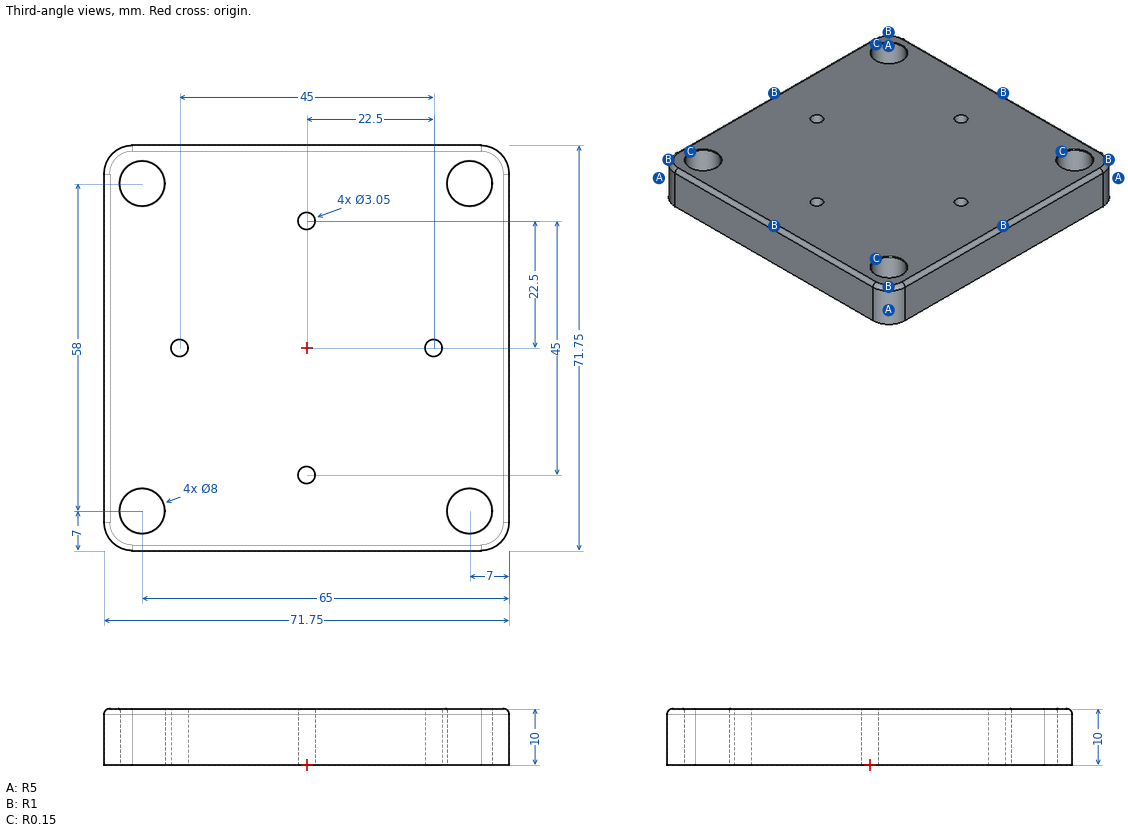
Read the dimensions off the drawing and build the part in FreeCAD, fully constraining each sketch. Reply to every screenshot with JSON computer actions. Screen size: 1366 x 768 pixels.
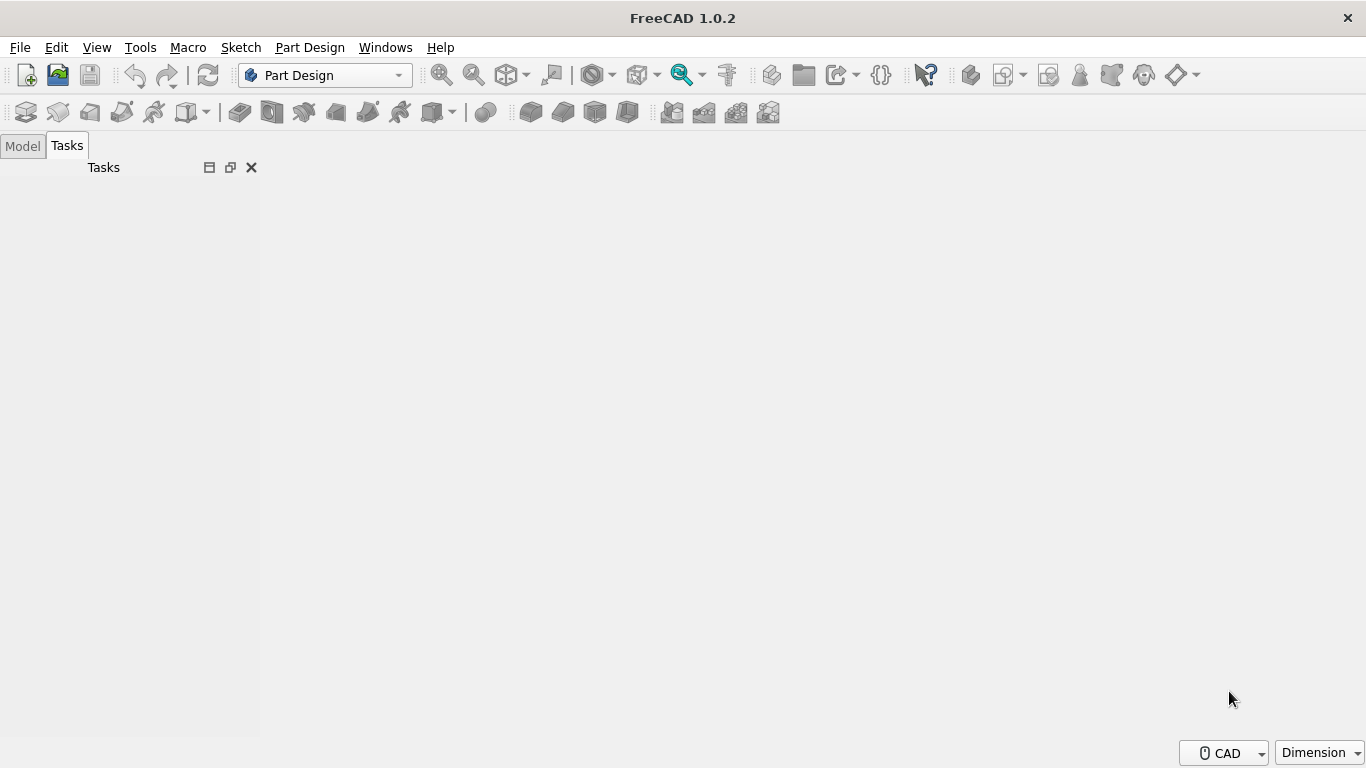
{"action": "left_click", "coordinate": [26, 76]}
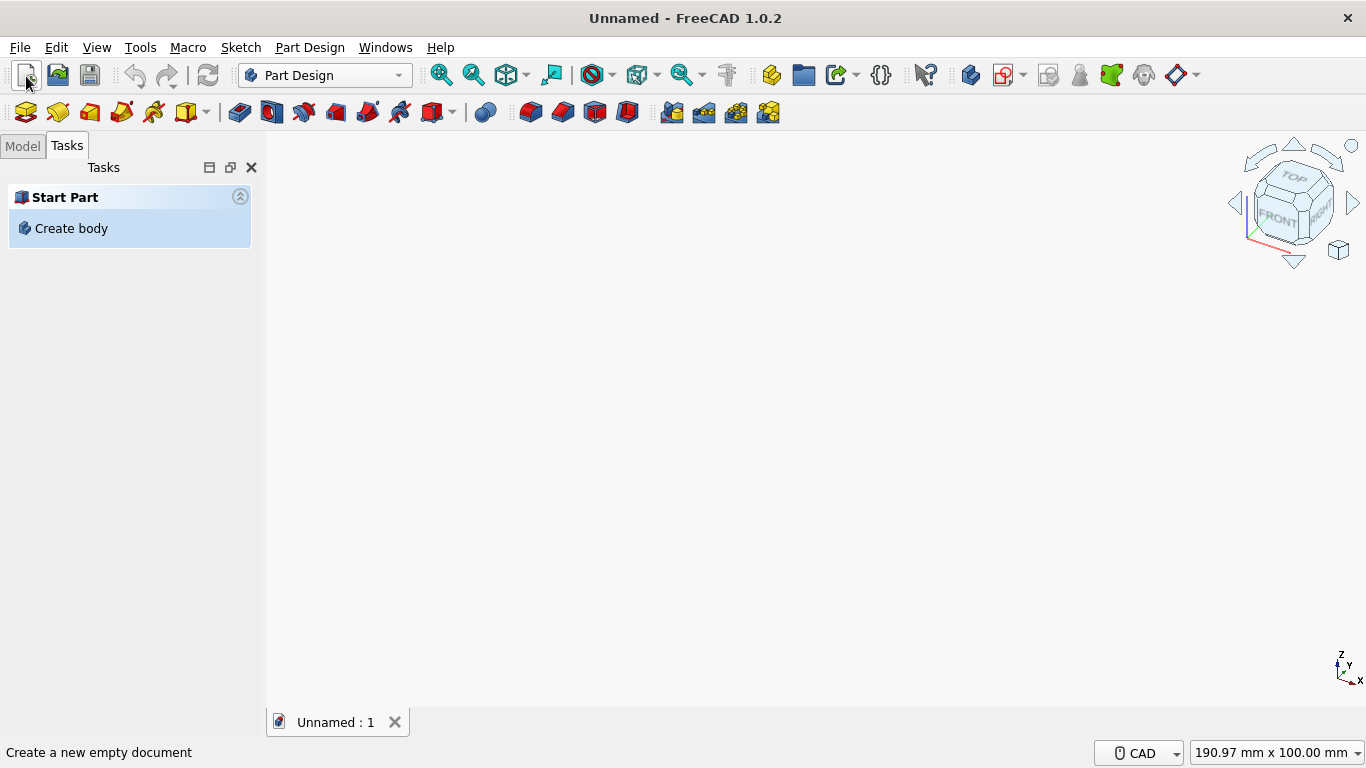
{"action": "left_click", "coordinate": [1004, 76]}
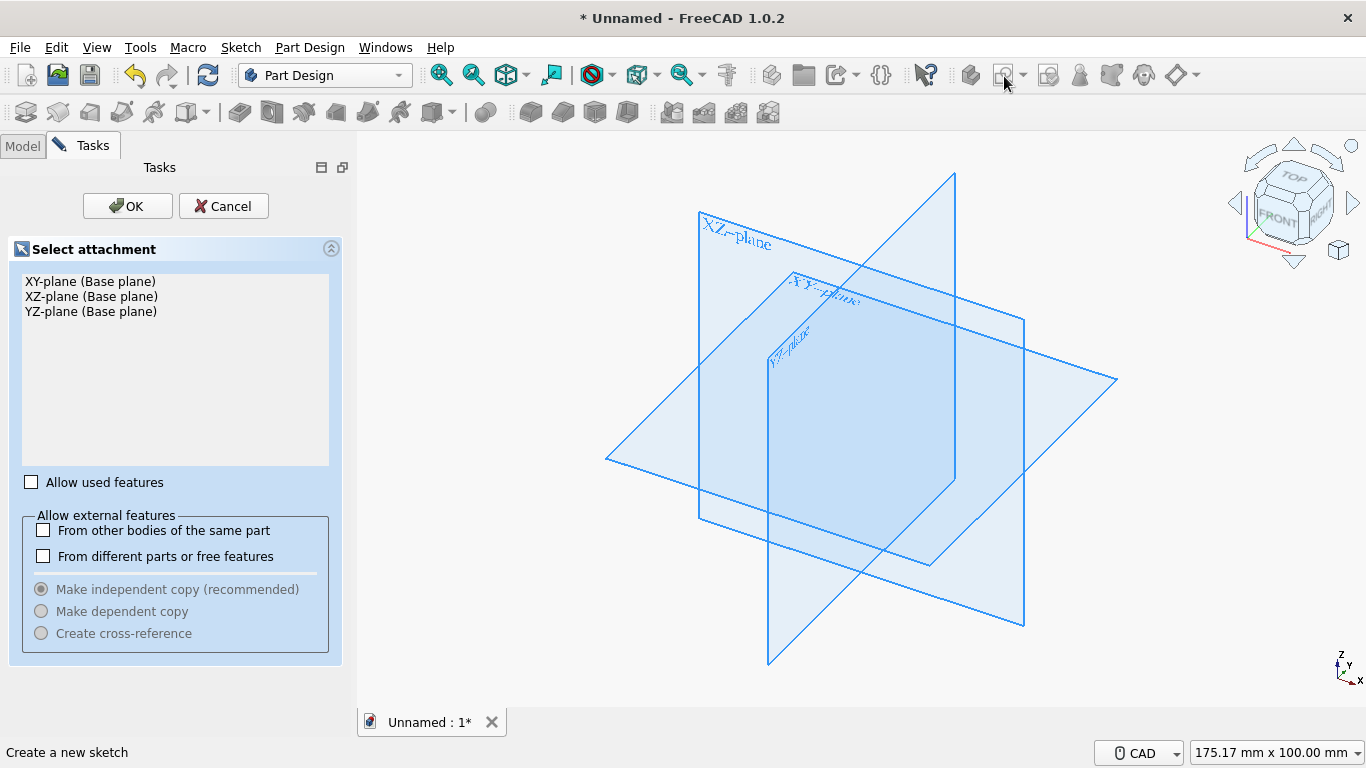
{"action": "left_click", "coordinate": [82, 282]}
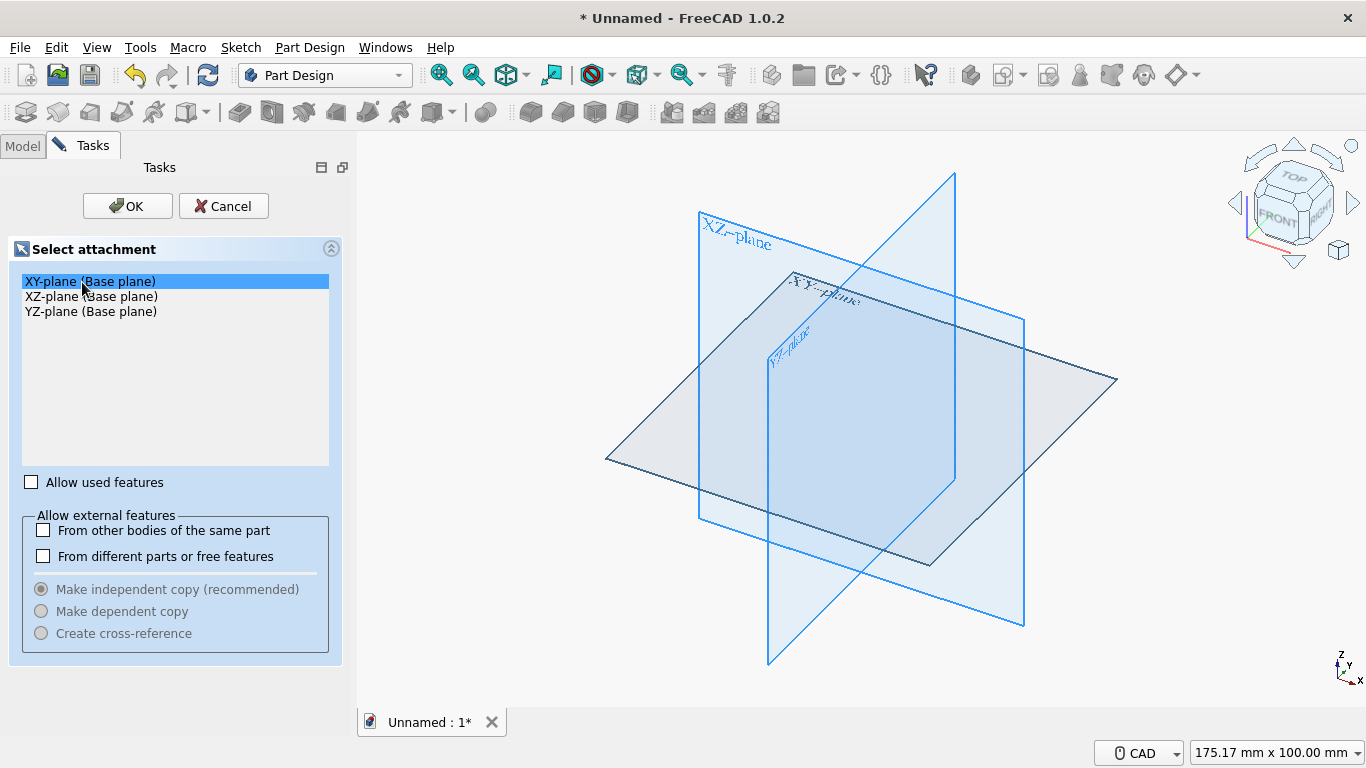
{"action": "left_click", "coordinate": [128, 206]}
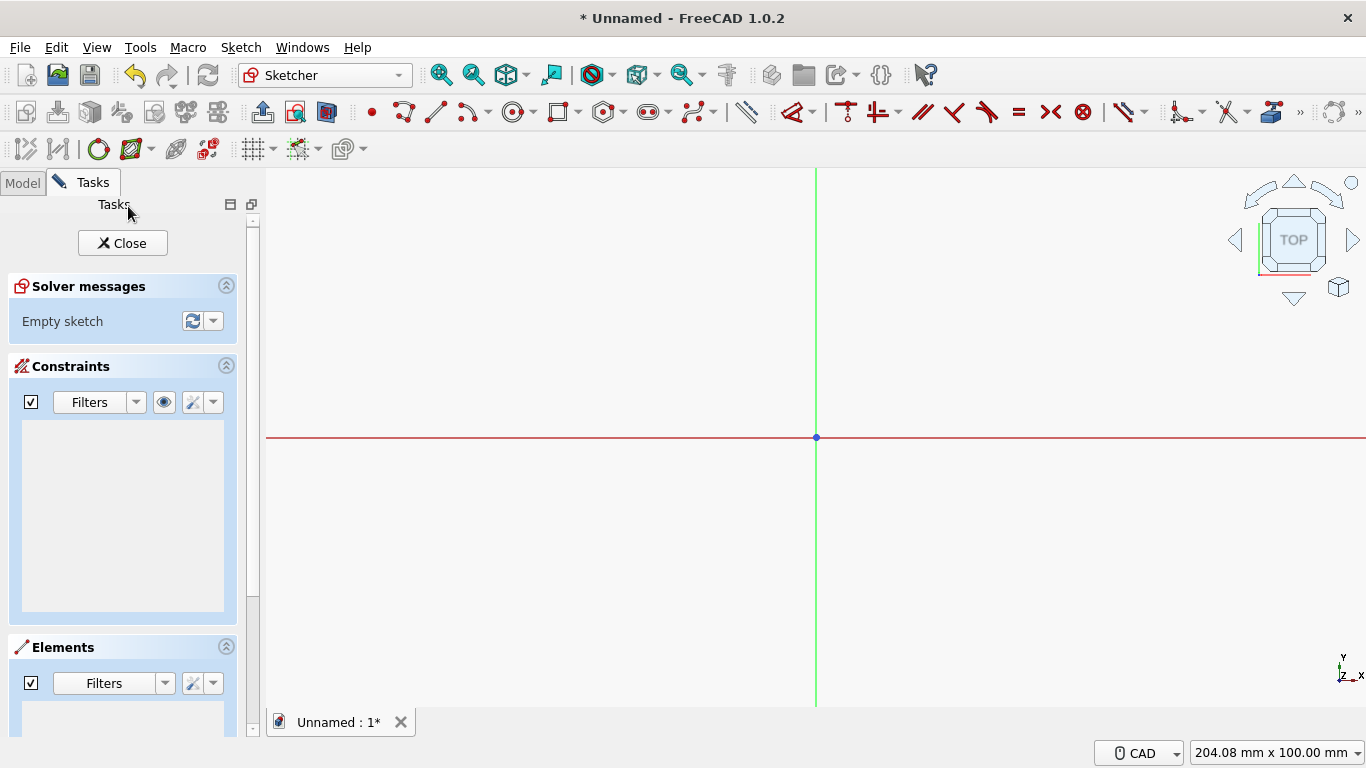
{"action": "key", "text": "g v"}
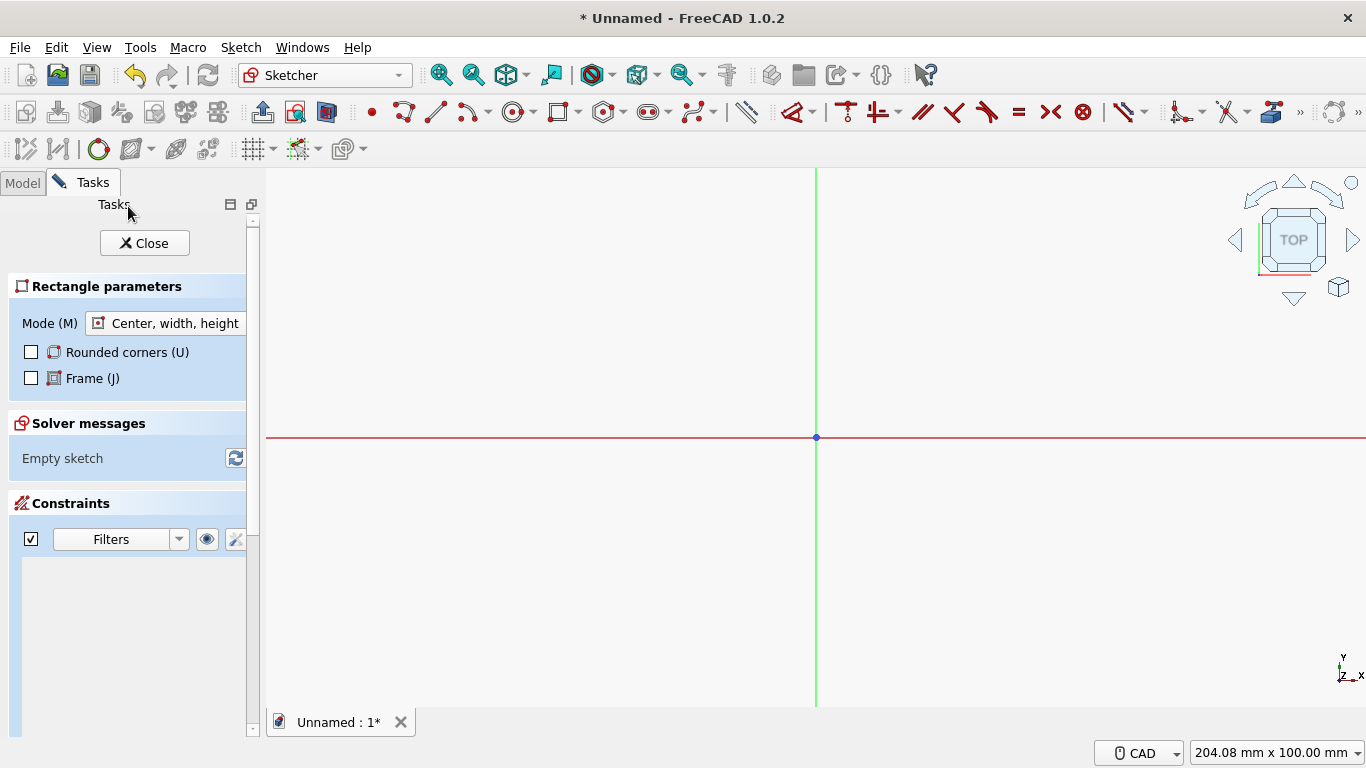
{"action": "left_click", "coordinate": [816, 438]}
{"action": "left_click", "coordinate": [1009, 244]}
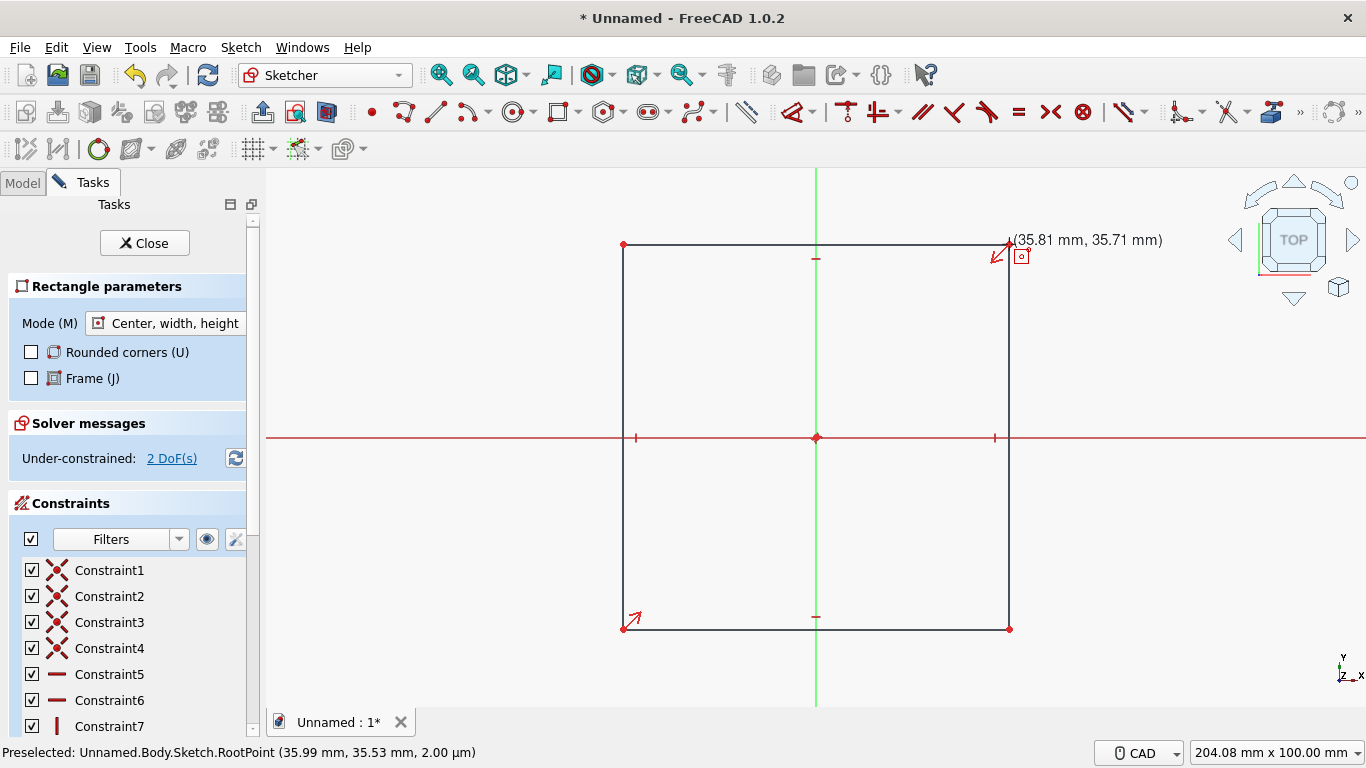
{"action": "left_click", "coordinate": [514, 112]}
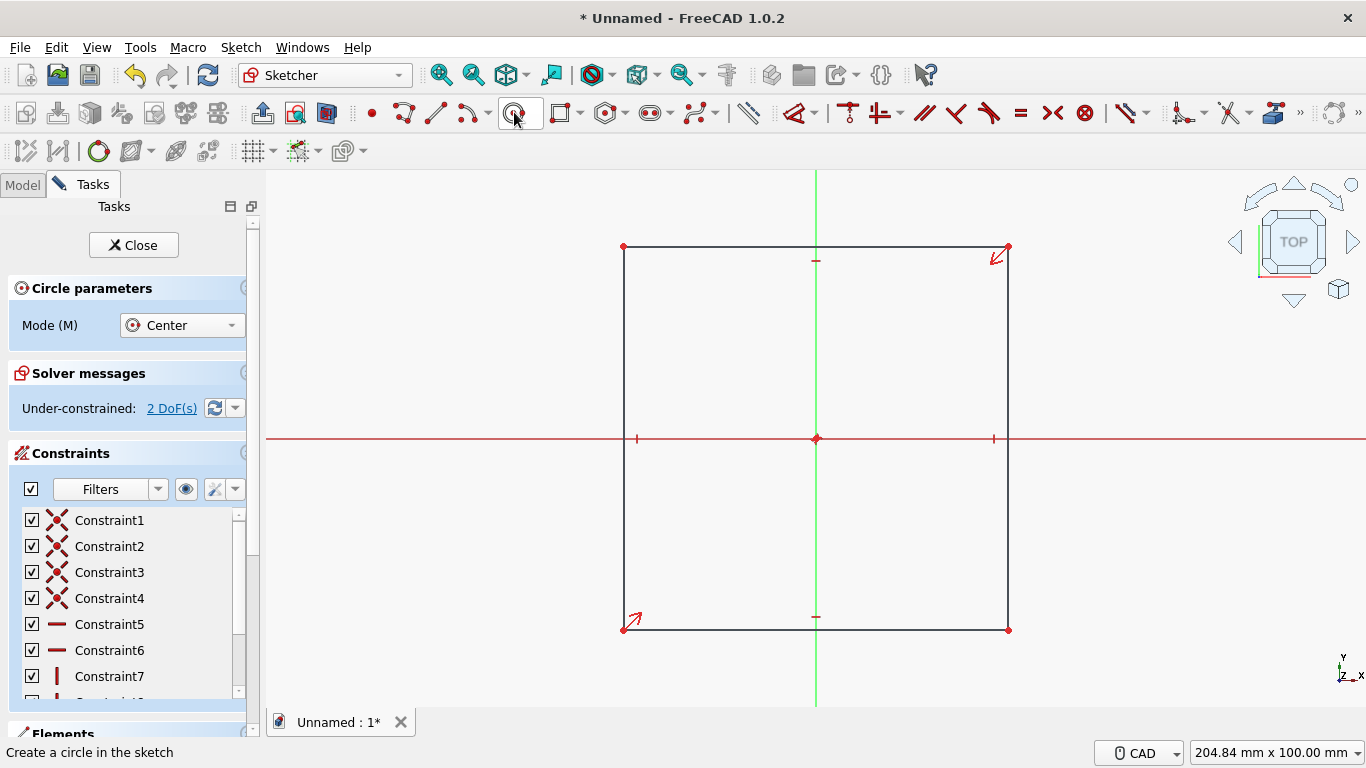
{"action": "left_click", "coordinate": [660, 594]}
{"action": "left_click", "coordinate": [675, 578]}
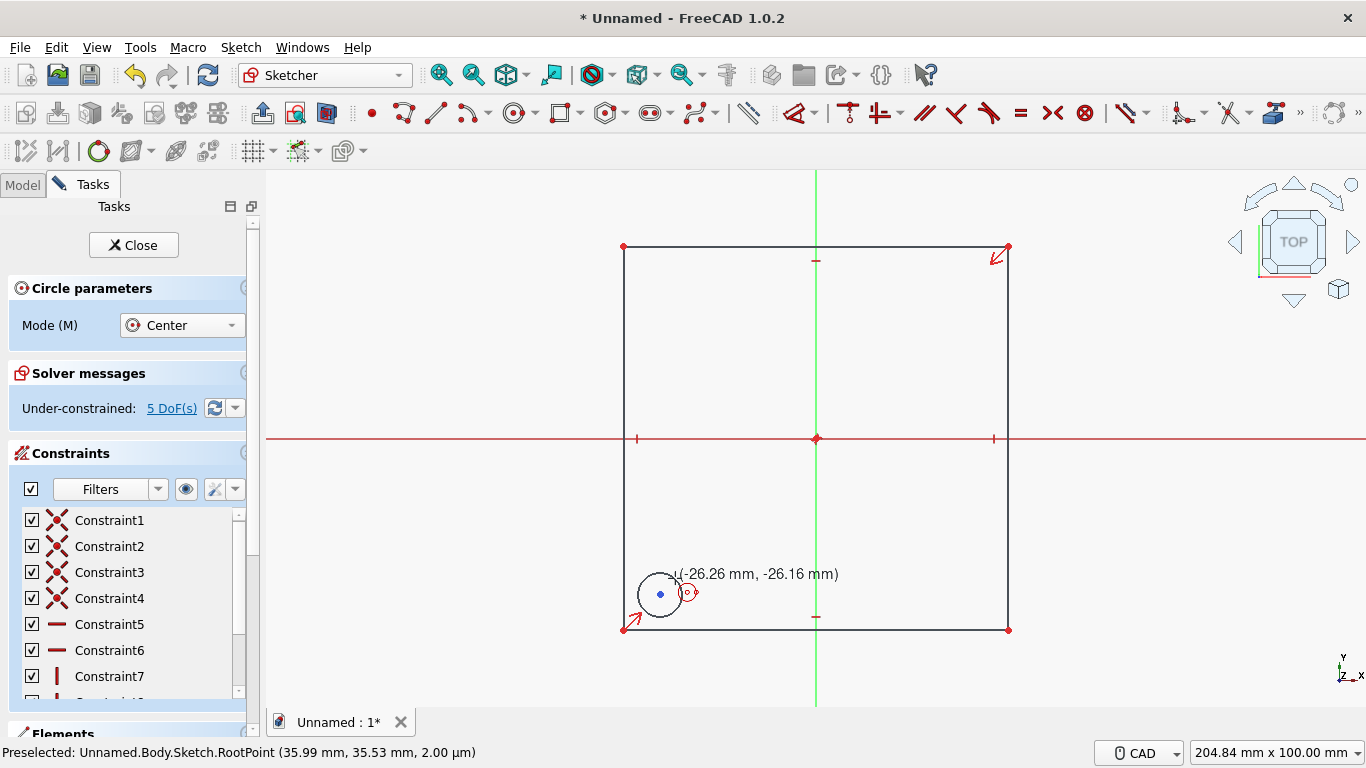
{"action": "left_click", "coordinate": [971, 594]}
{"action": "left_click", "coordinate": [986, 578]}